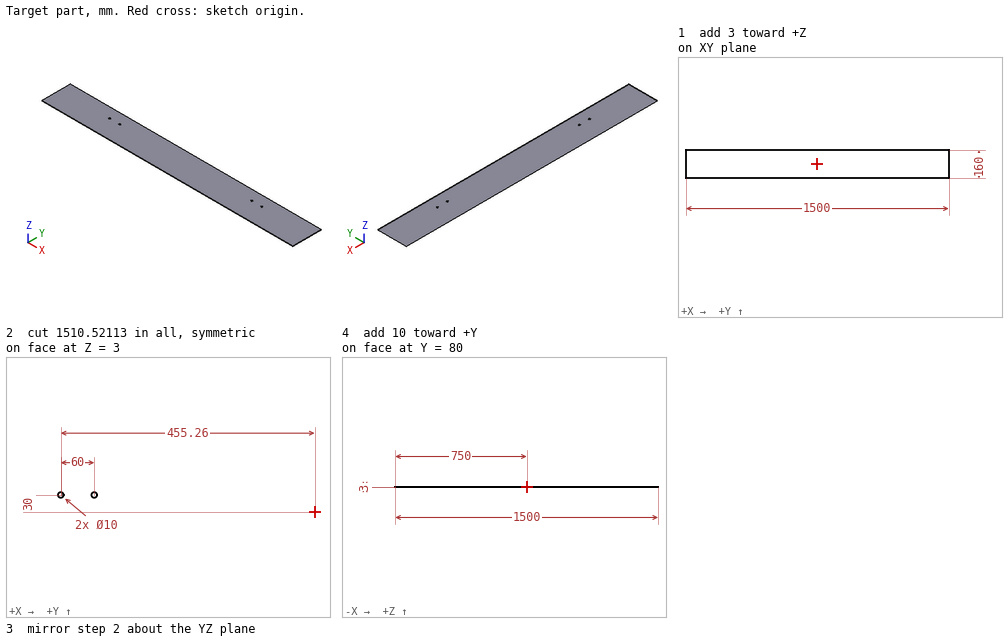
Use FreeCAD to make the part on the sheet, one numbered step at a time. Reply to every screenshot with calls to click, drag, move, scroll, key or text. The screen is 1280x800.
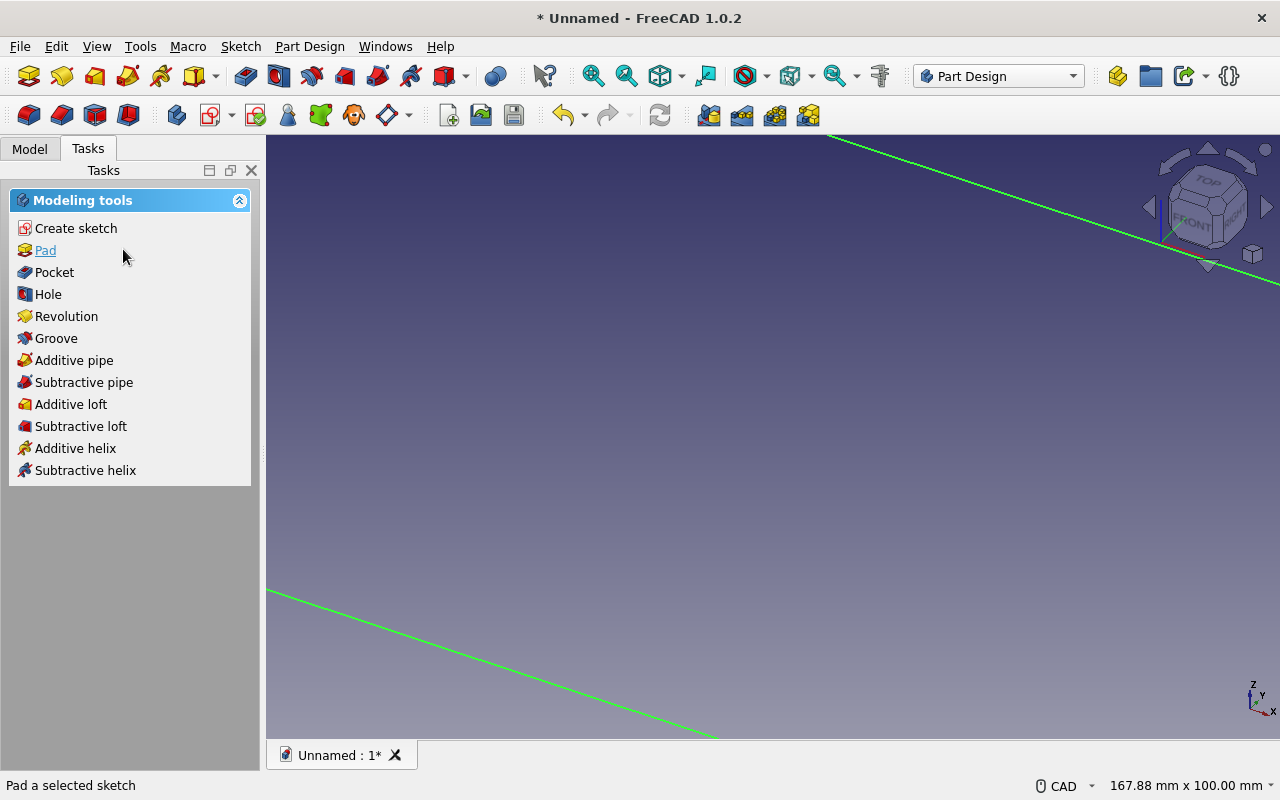
click(29, 76)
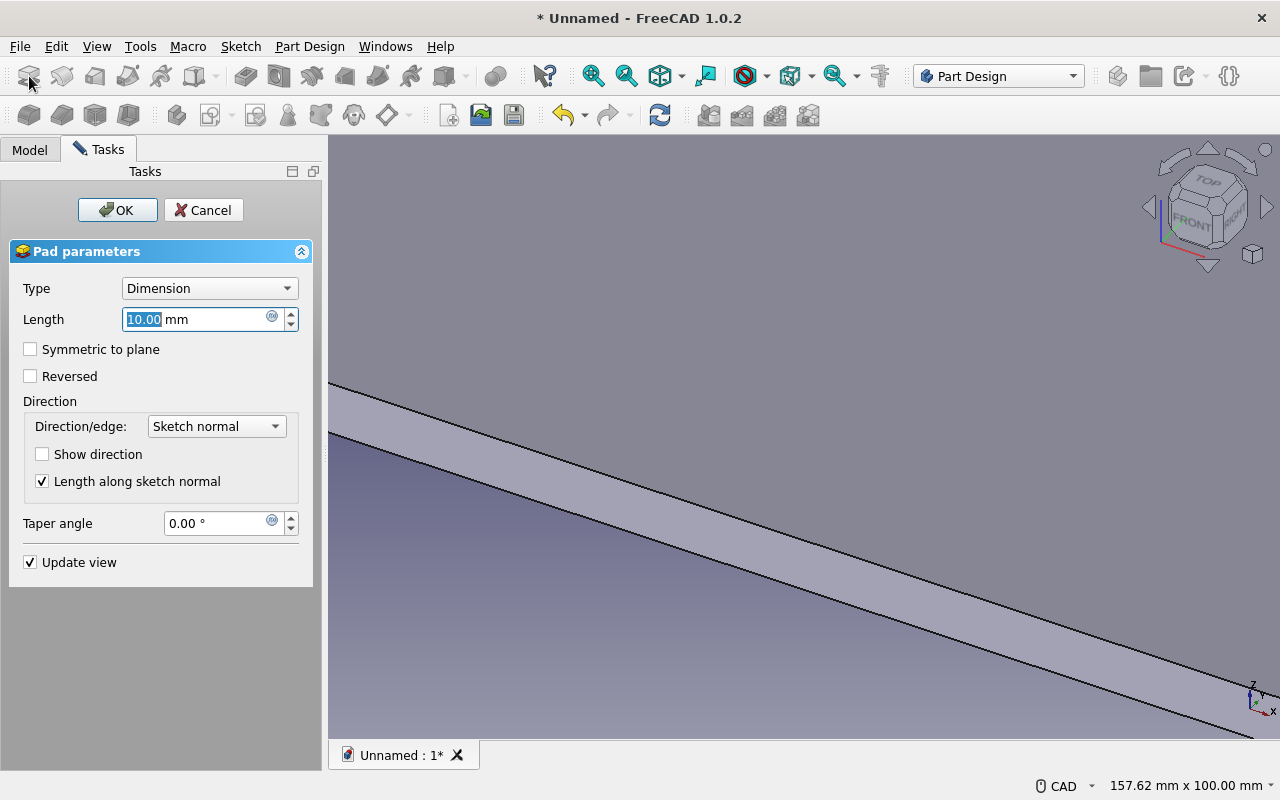
text(3)
key(Tab)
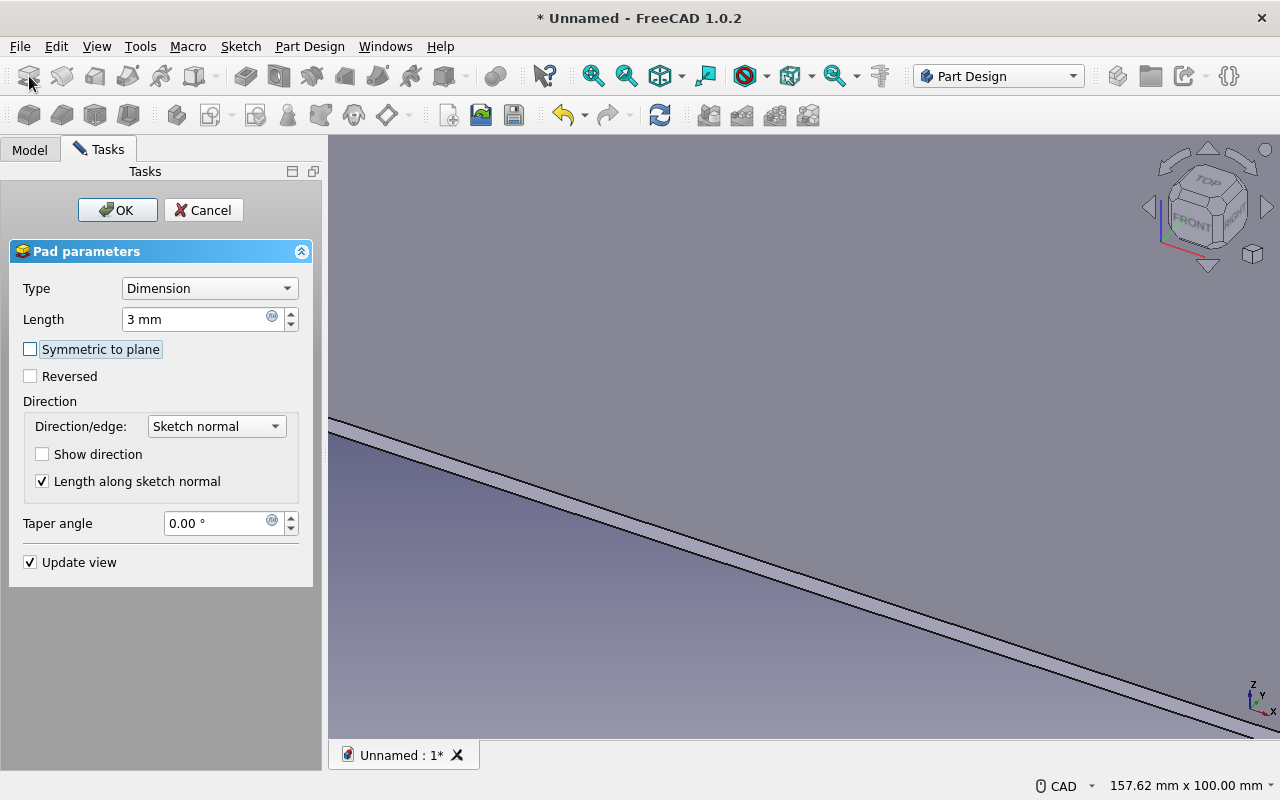
click(118, 210)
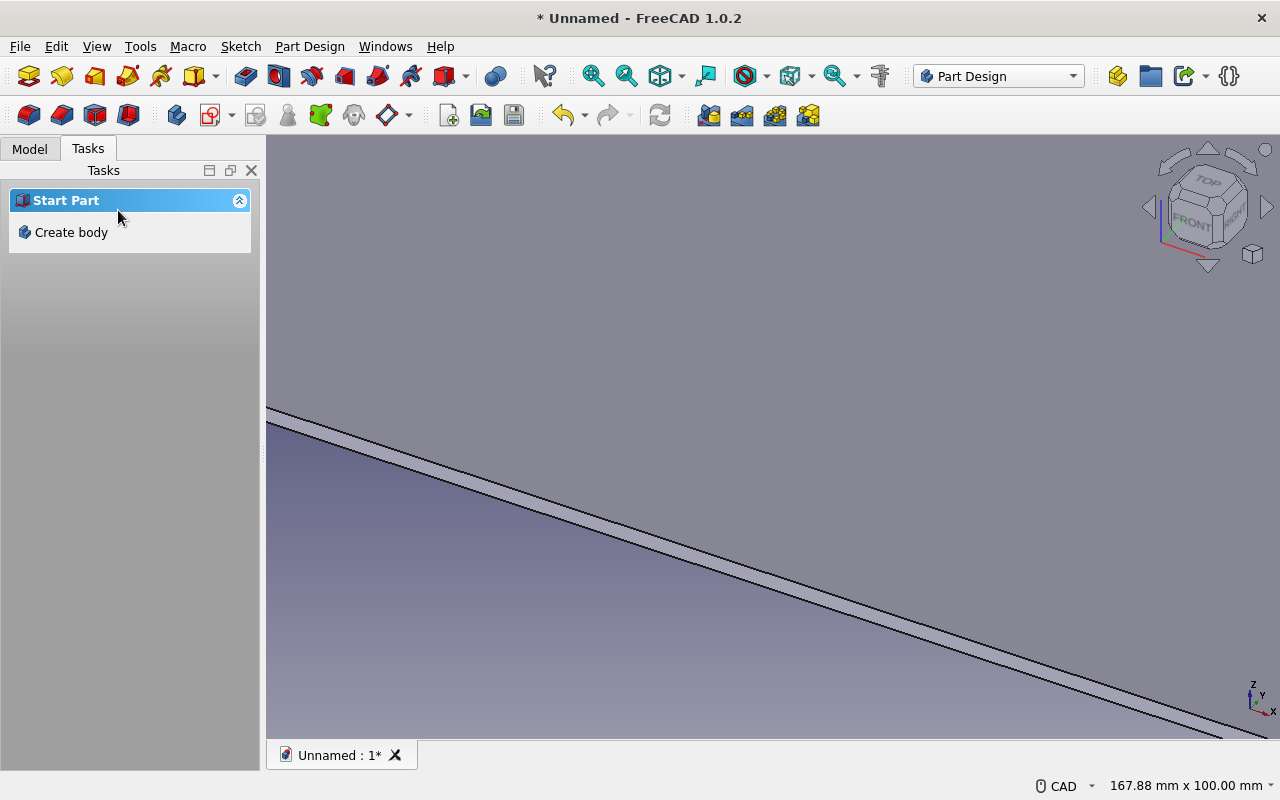
click(594, 76)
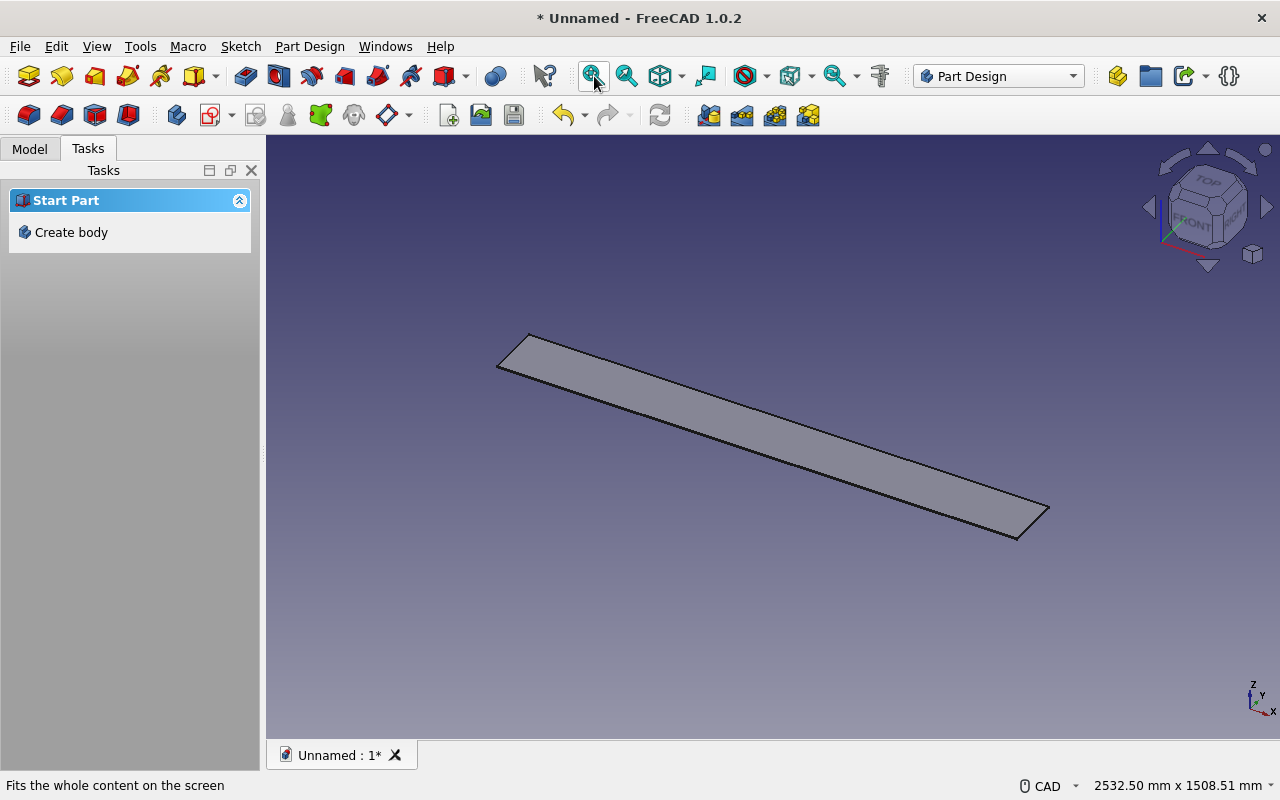
click(996, 509)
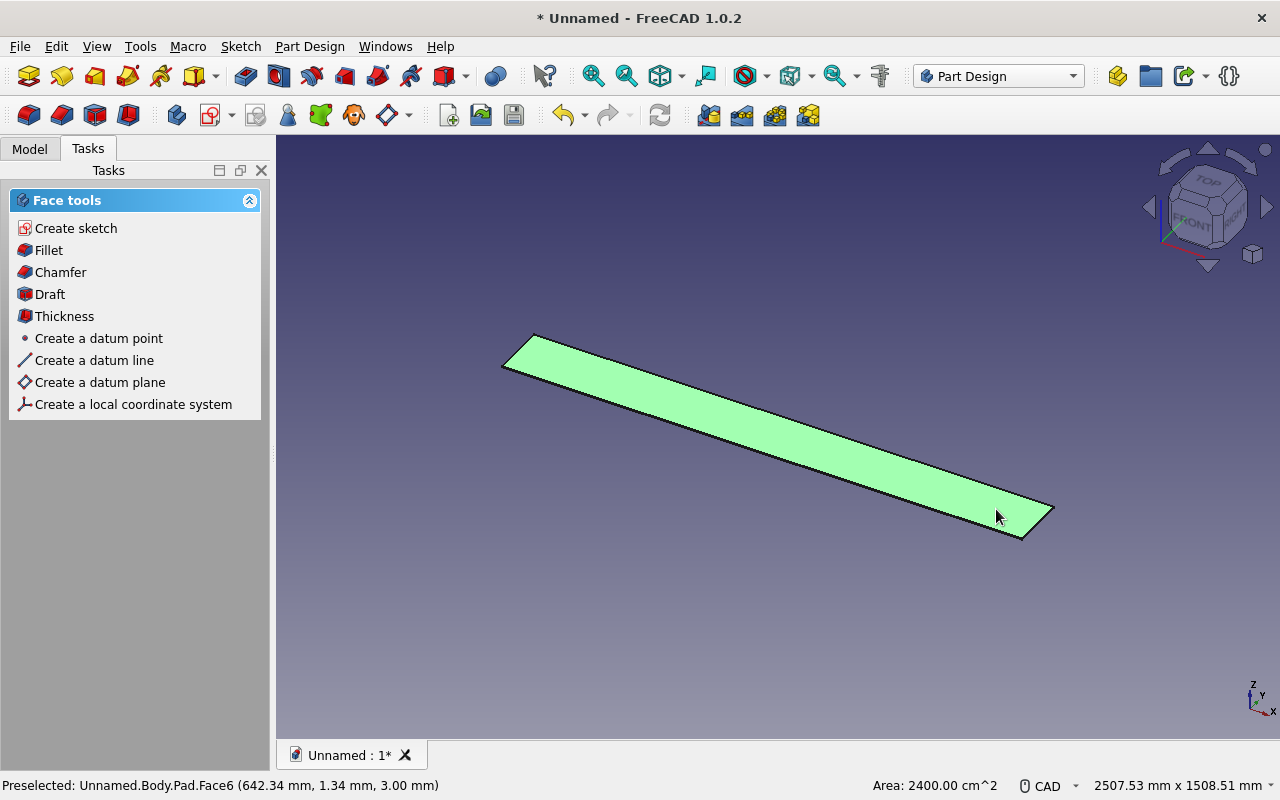
click(210, 116)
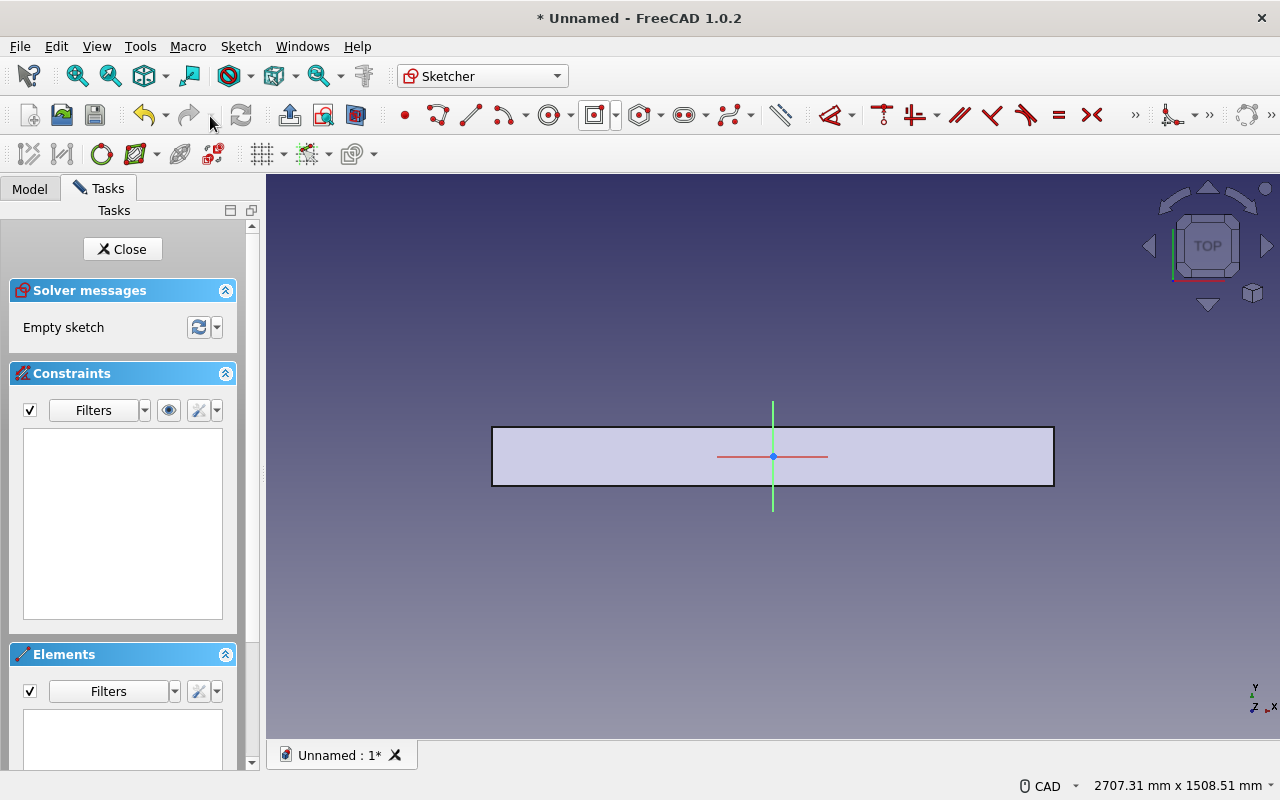
scroll(609, 445, up, 15)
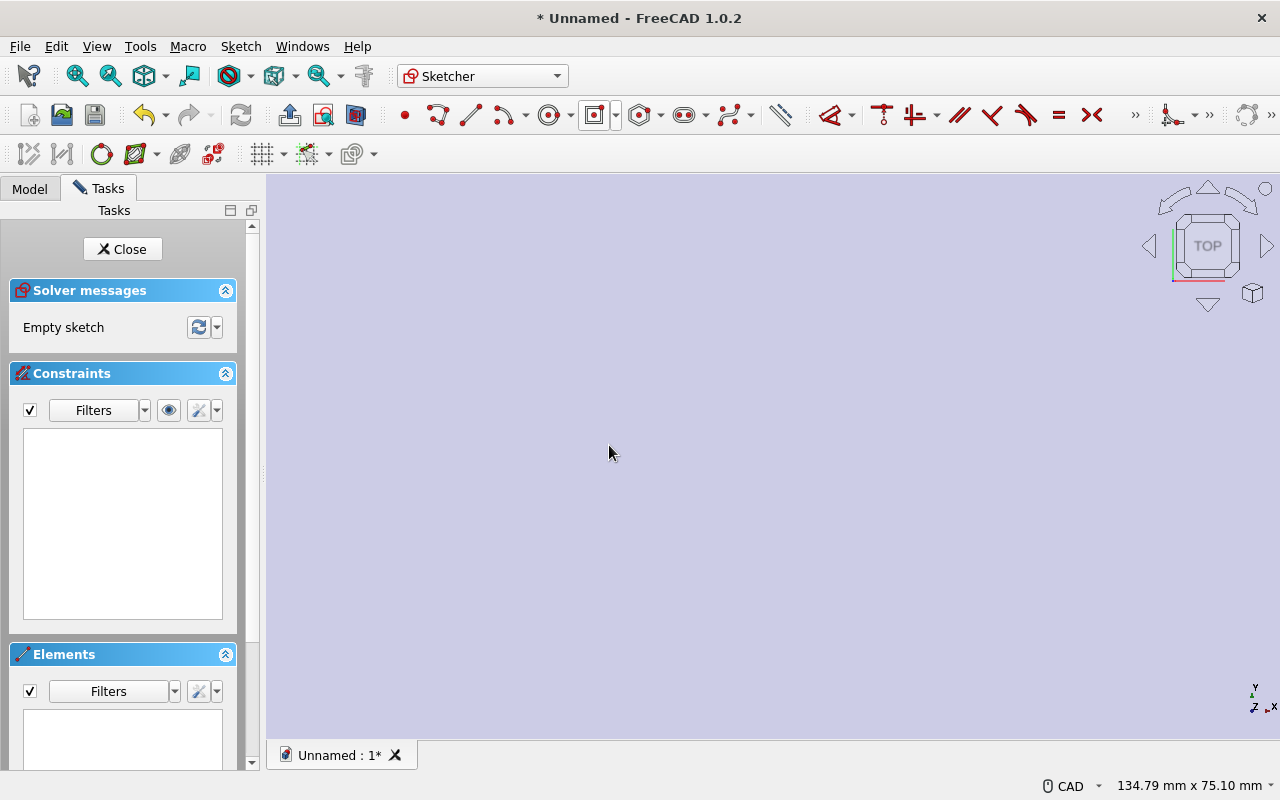
click(548, 116)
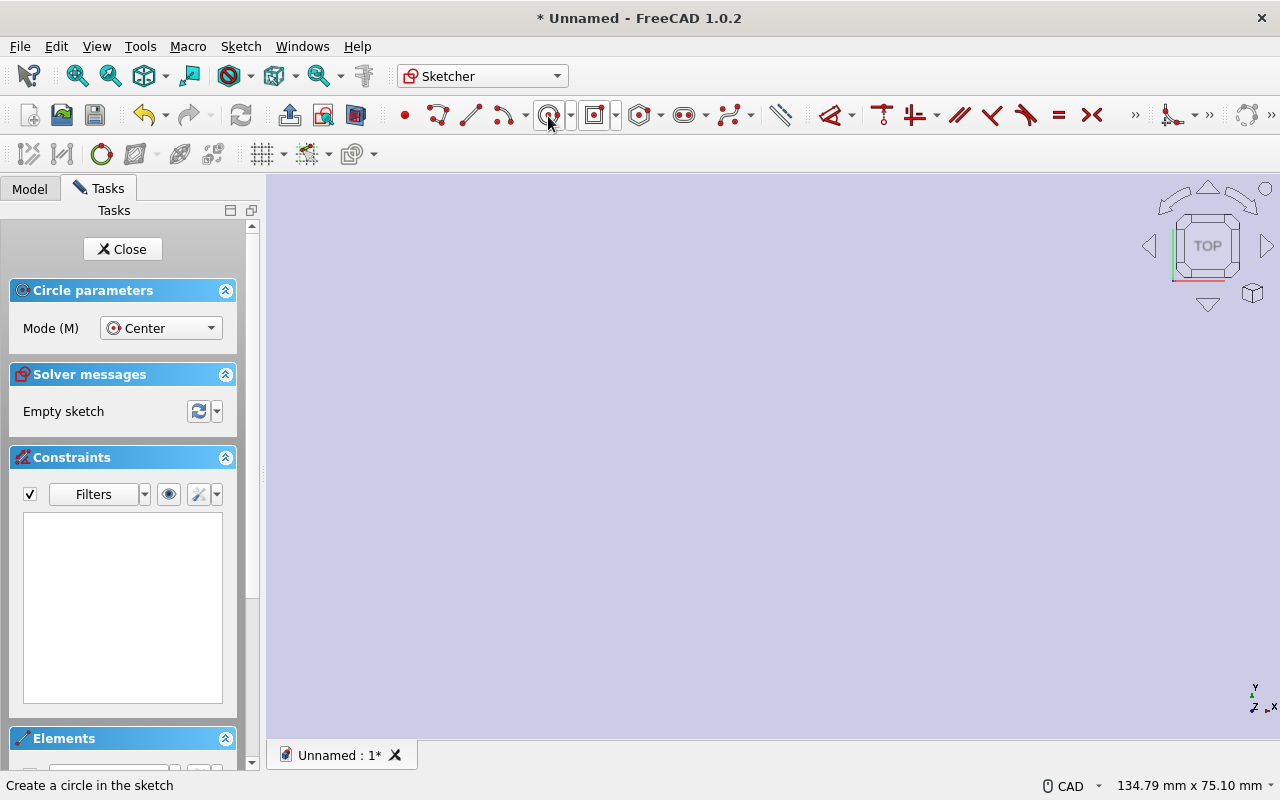
click(472, 441)
move(498, 415)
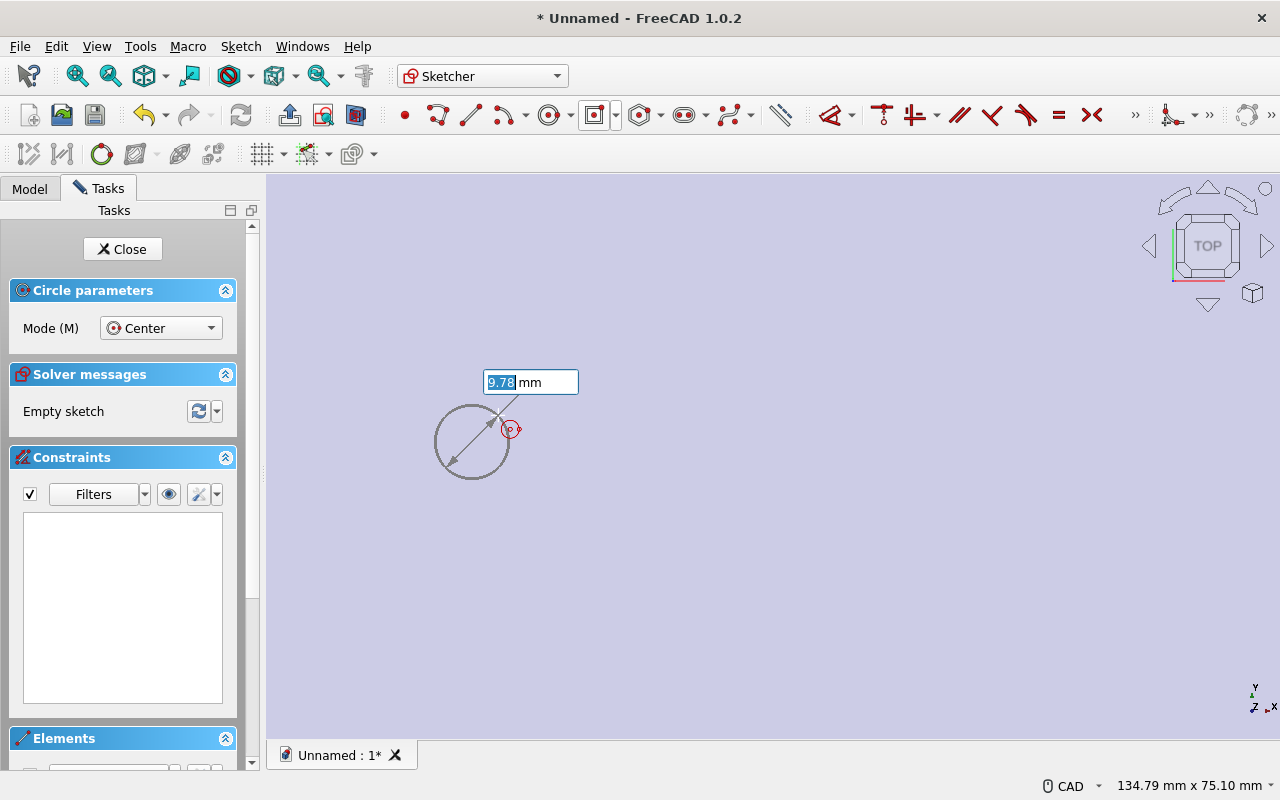
text(10)
key(Return)